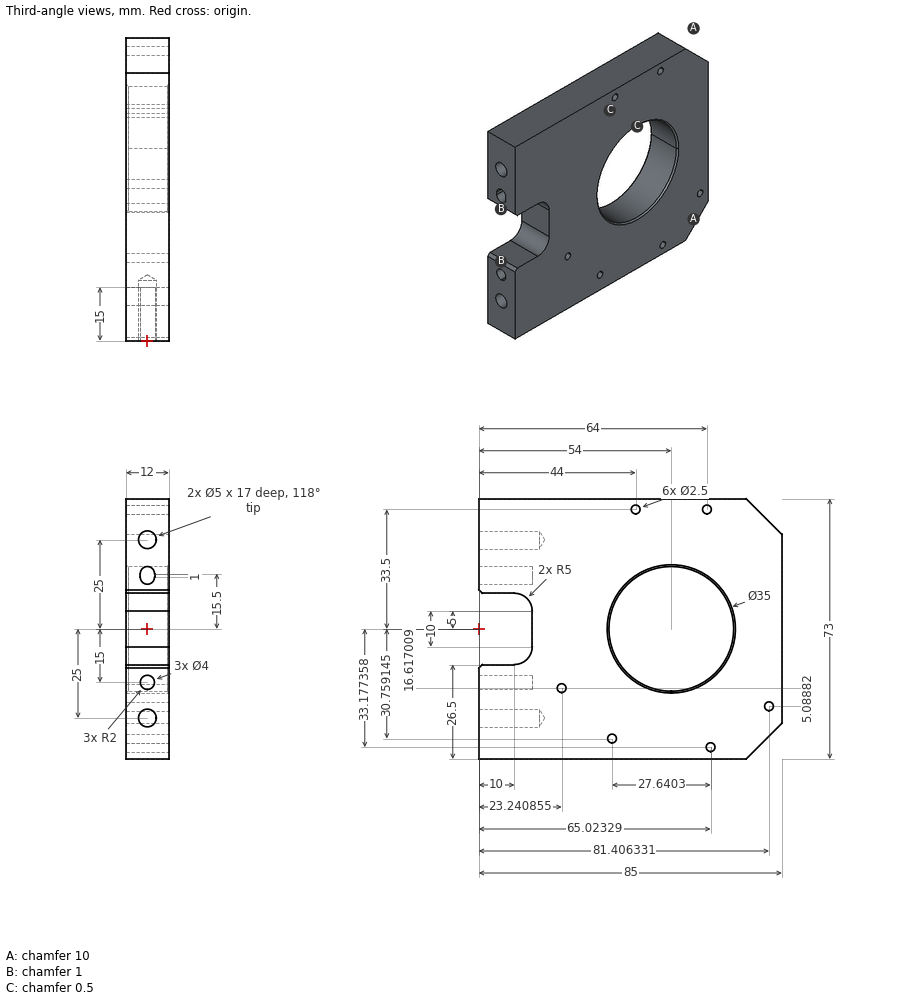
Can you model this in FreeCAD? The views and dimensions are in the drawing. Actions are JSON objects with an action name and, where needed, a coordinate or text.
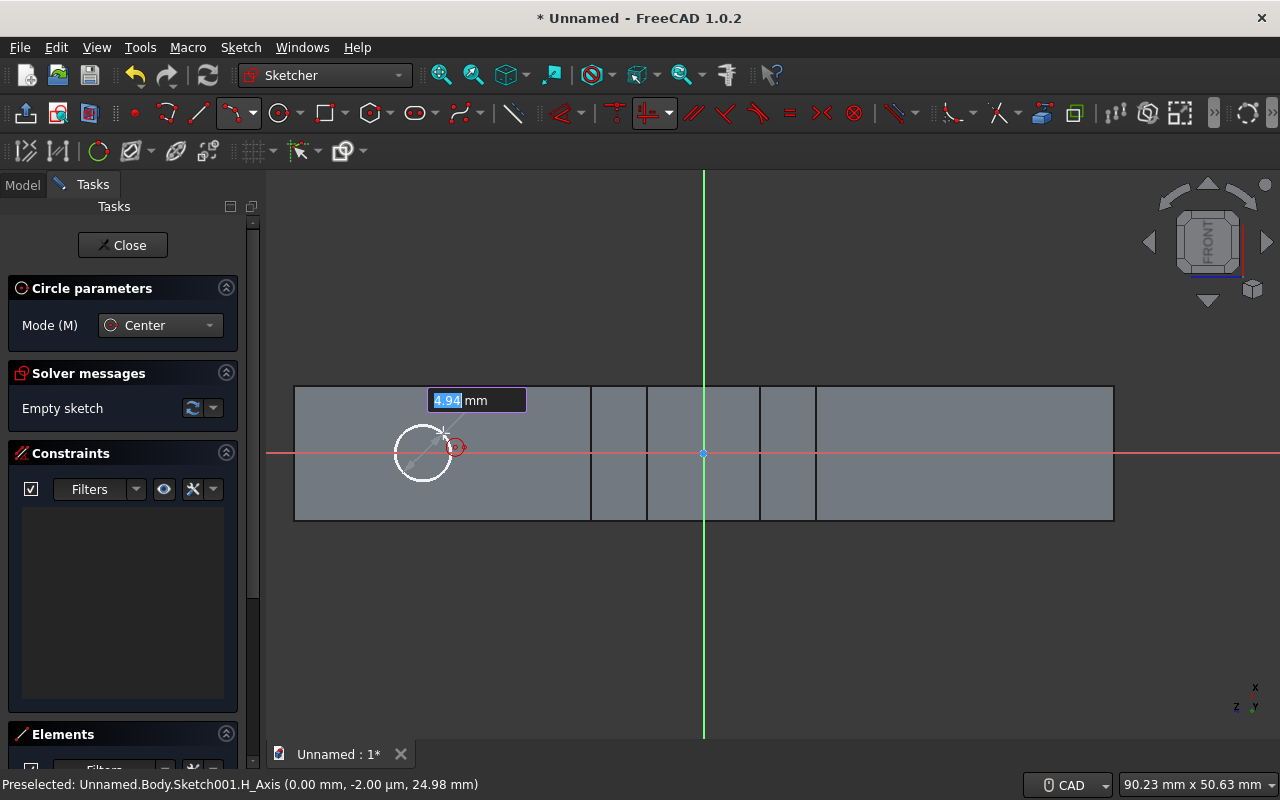
{"action": "type", "text": "5"}
{"action": "key", "text": "Return"}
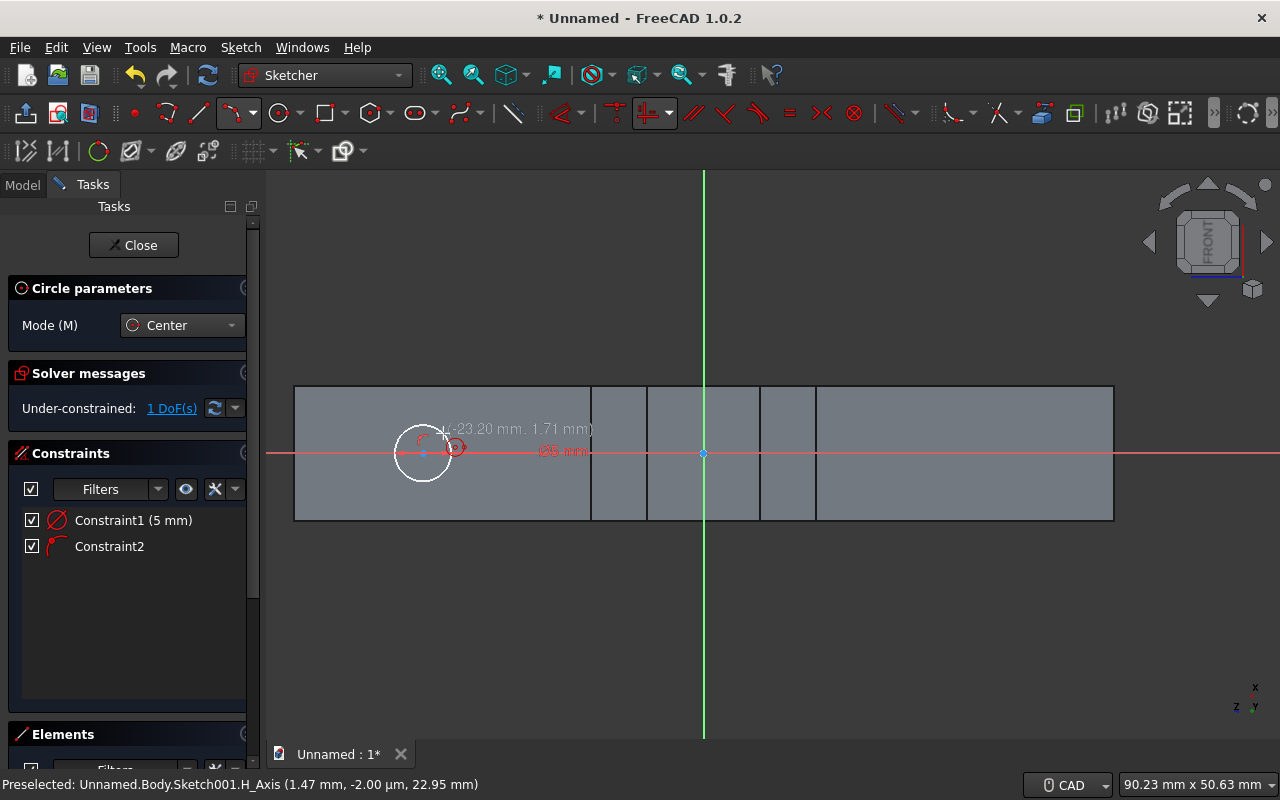
{"action": "left_click", "coordinate": [985, 453]}
{"action": "mouse_move", "coordinate": [1004, 433]}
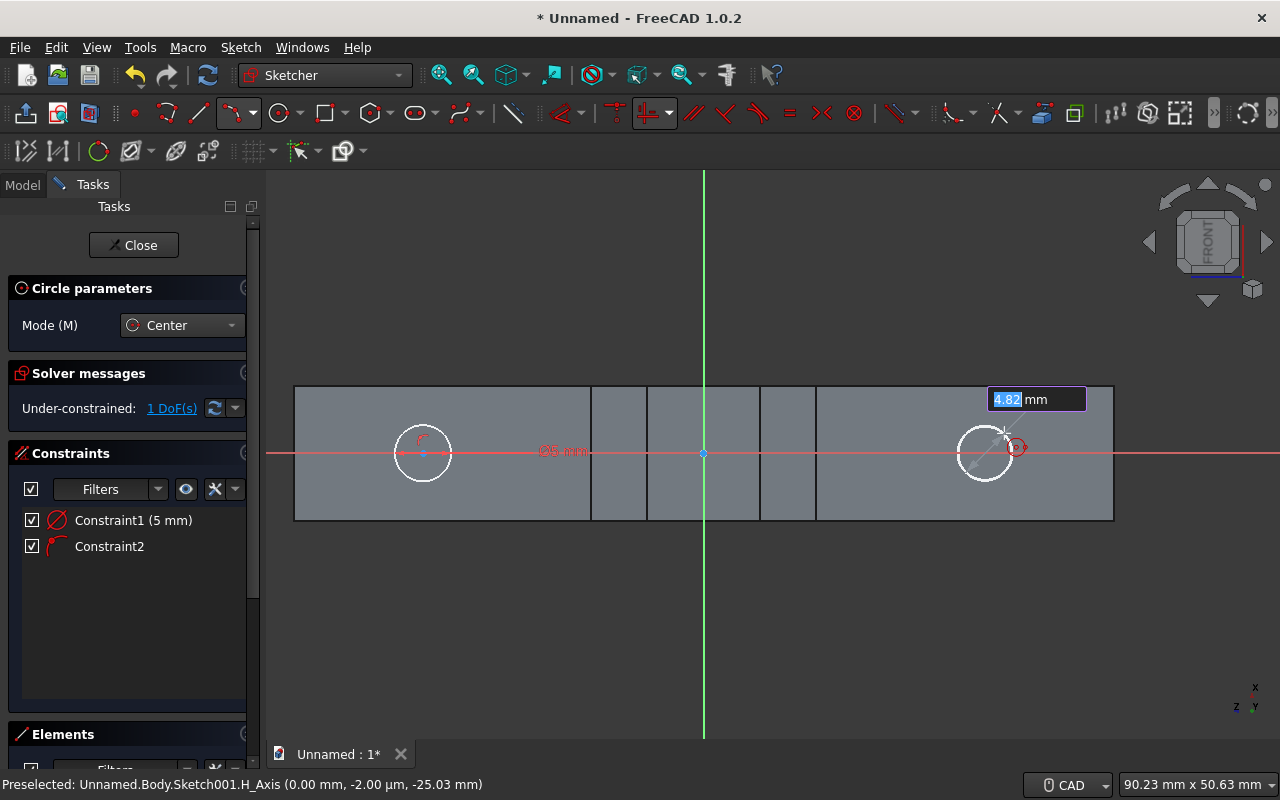
{"action": "type", "text": "5"}
{"action": "key", "text": "Return"}
{"action": "key", "text": "Escape"}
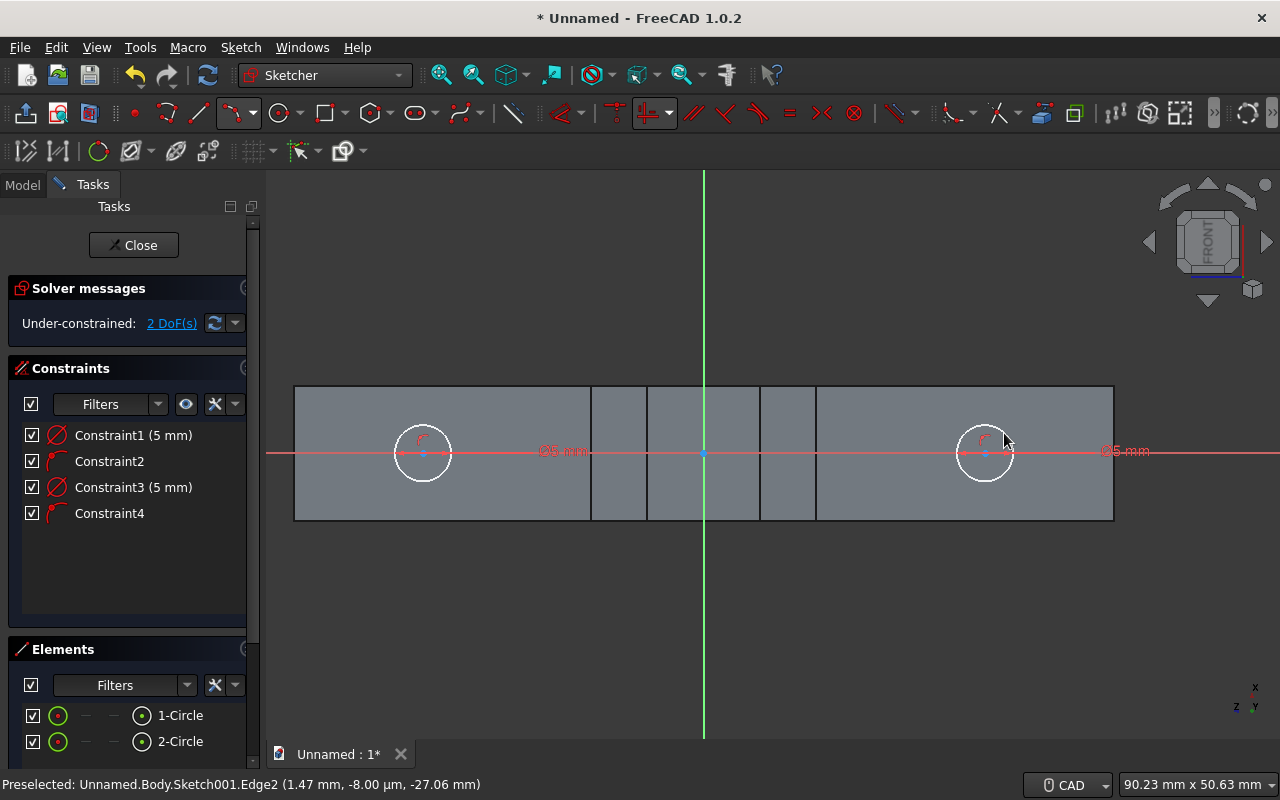
{"action": "left_click", "coordinate": [560, 114]}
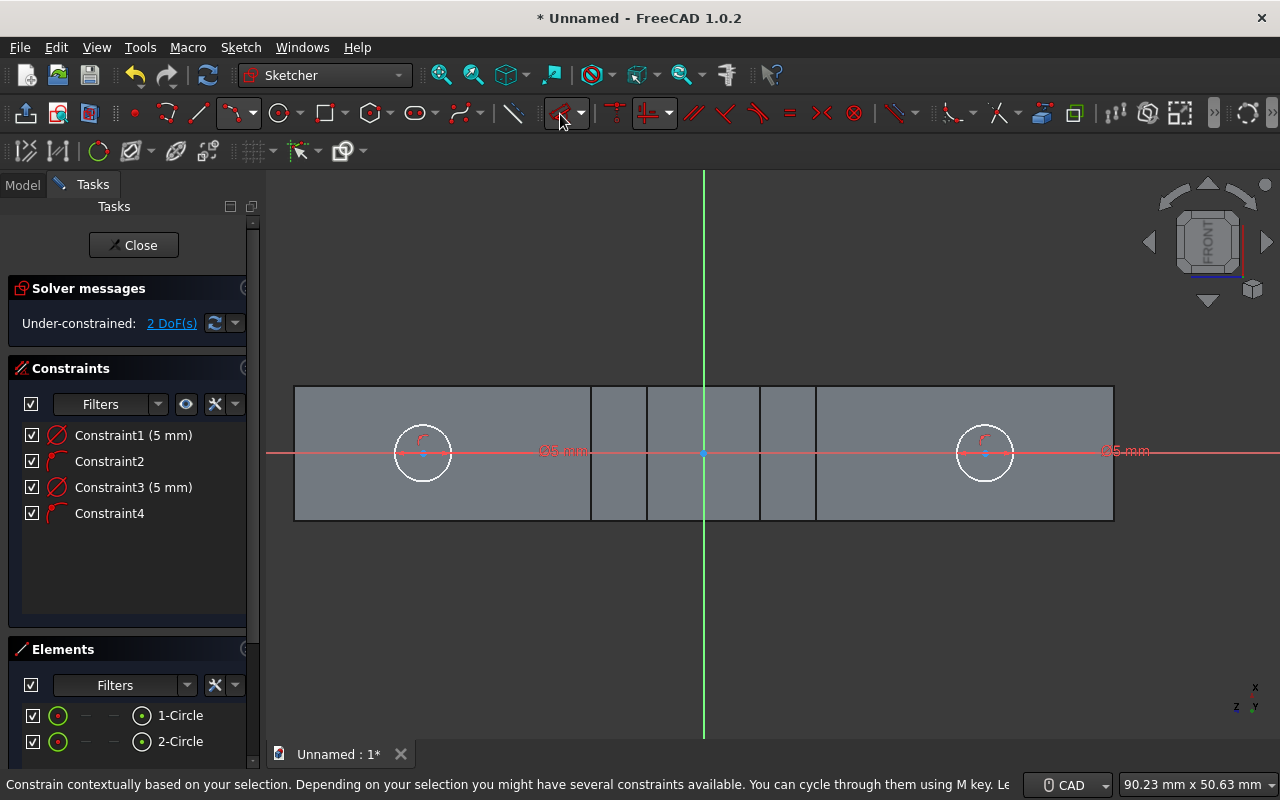
{"action": "left_click", "coordinate": [423, 453]}
{"action": "left_click", "coordinate": [563, 487]}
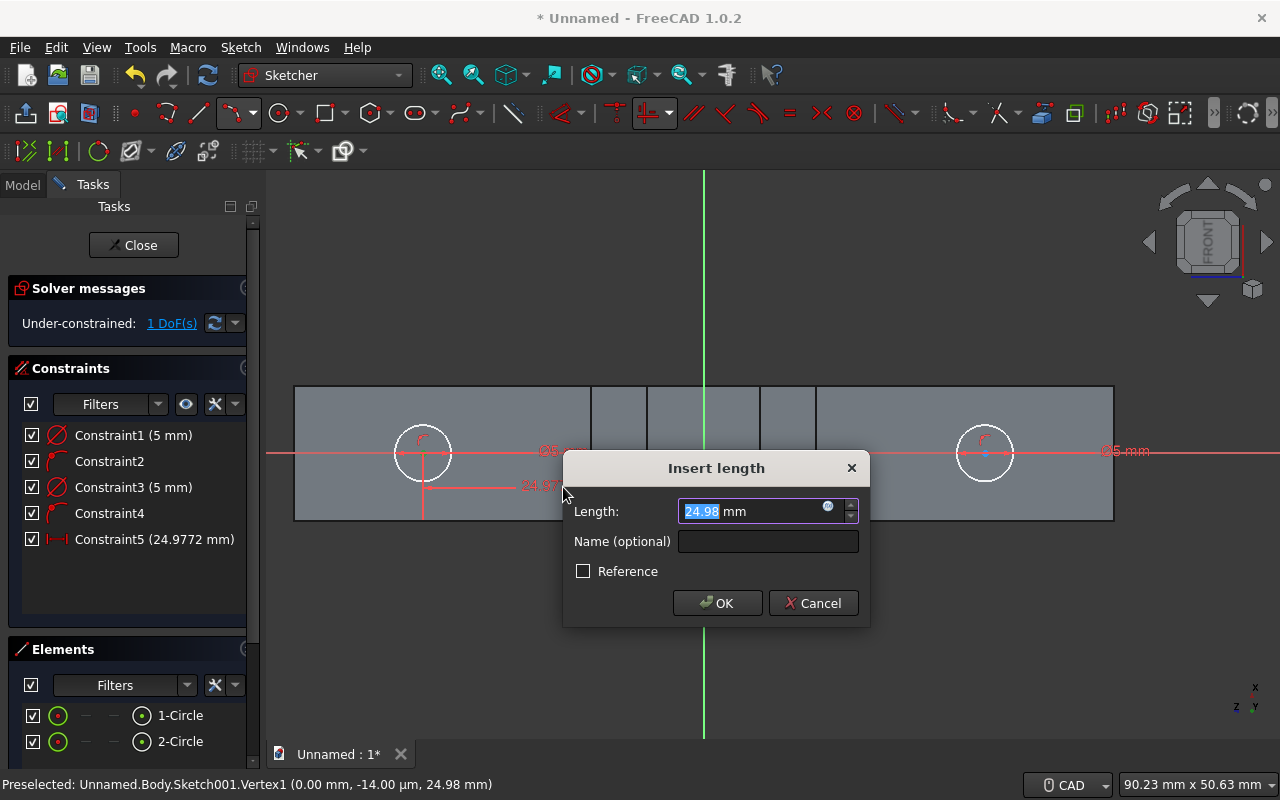
{"action": "type", "text": "25"}
{"action": "key", "text": "Return"}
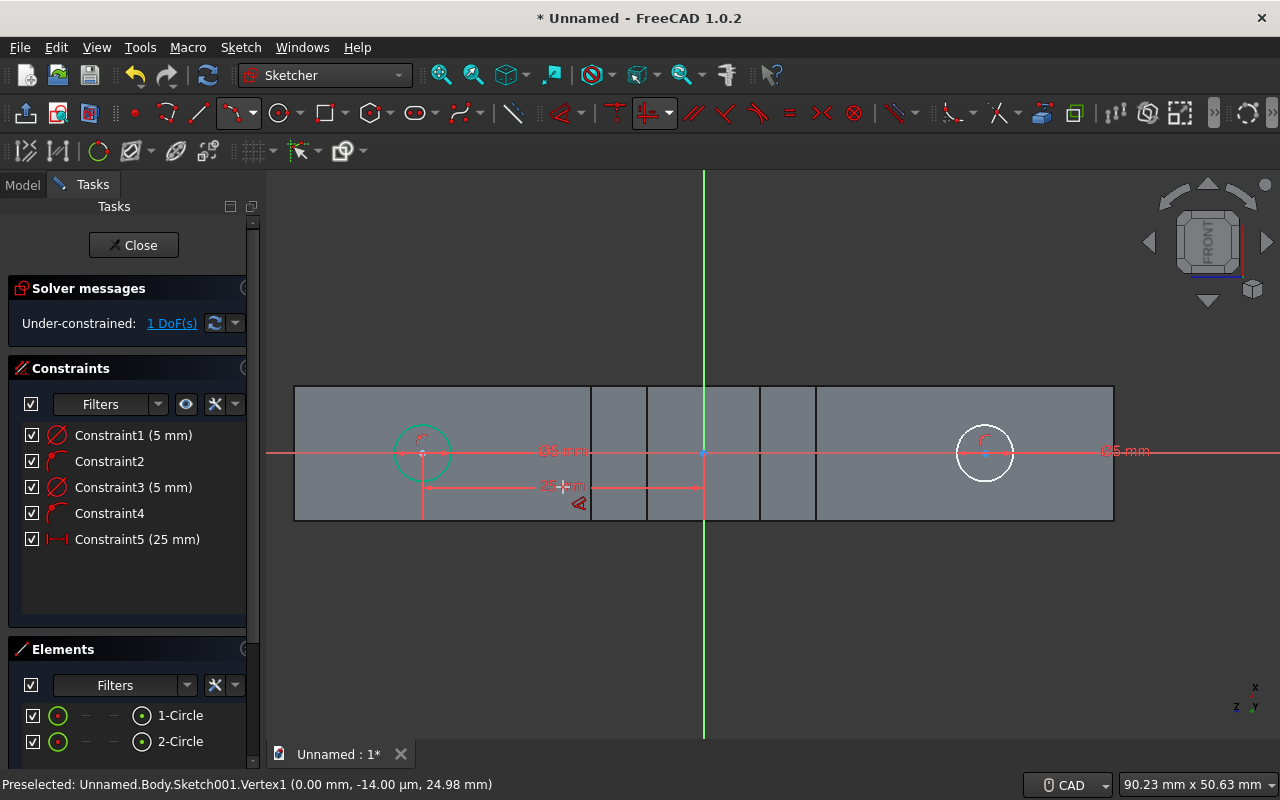
{"action": "left_click", "coordinate": [985, 453]}
{"action": "left_click", "coordinate": [844, 487]}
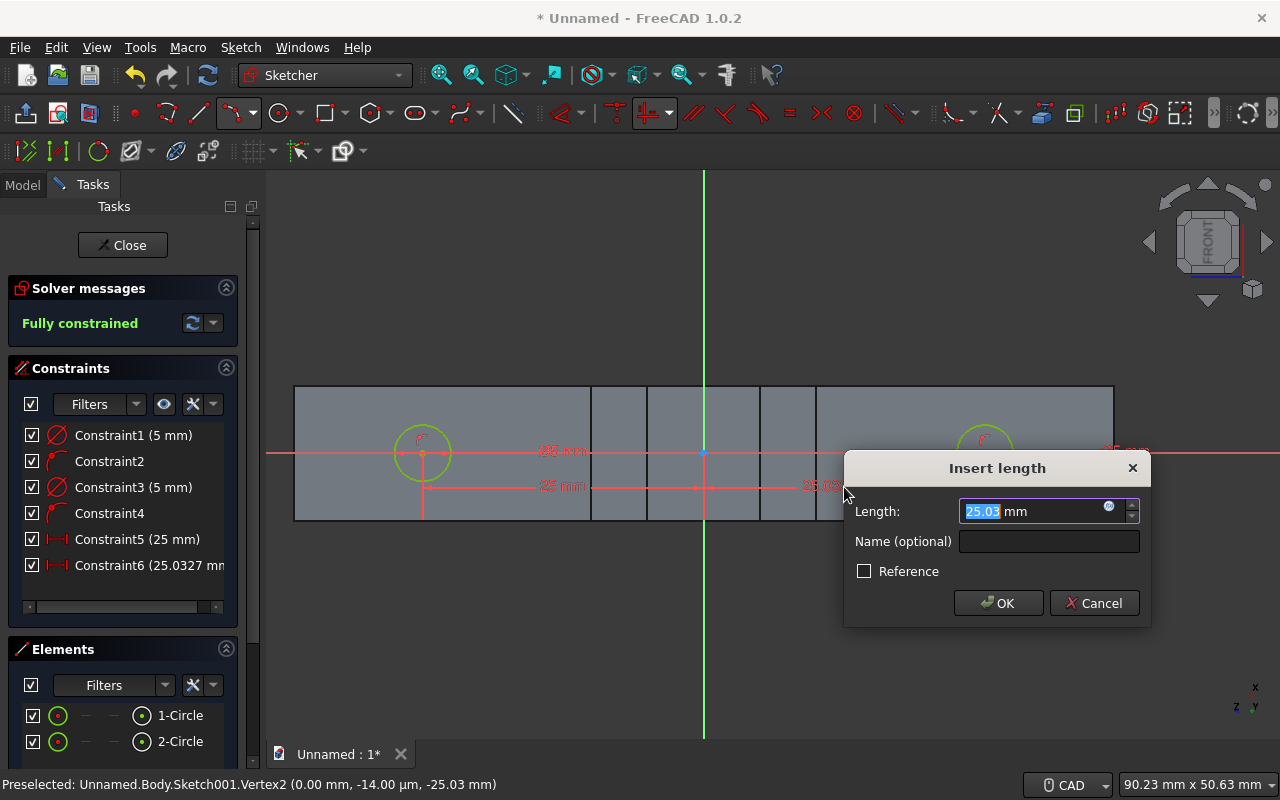
{"action": "type", "text": "25"}
{"action": "key", "text": "Return"}
{"action": "key", "text": "Escape"}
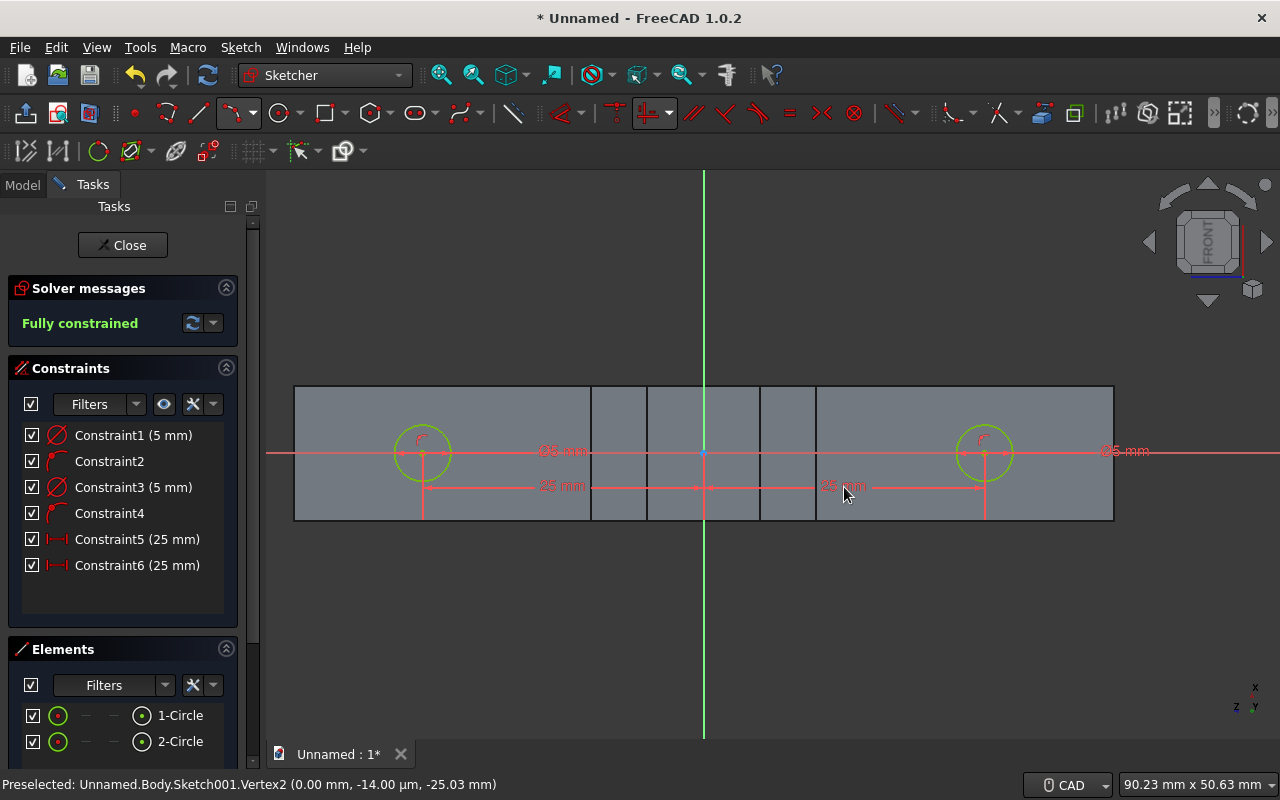
{"action": "left_click", "coordinate": [123, 245]}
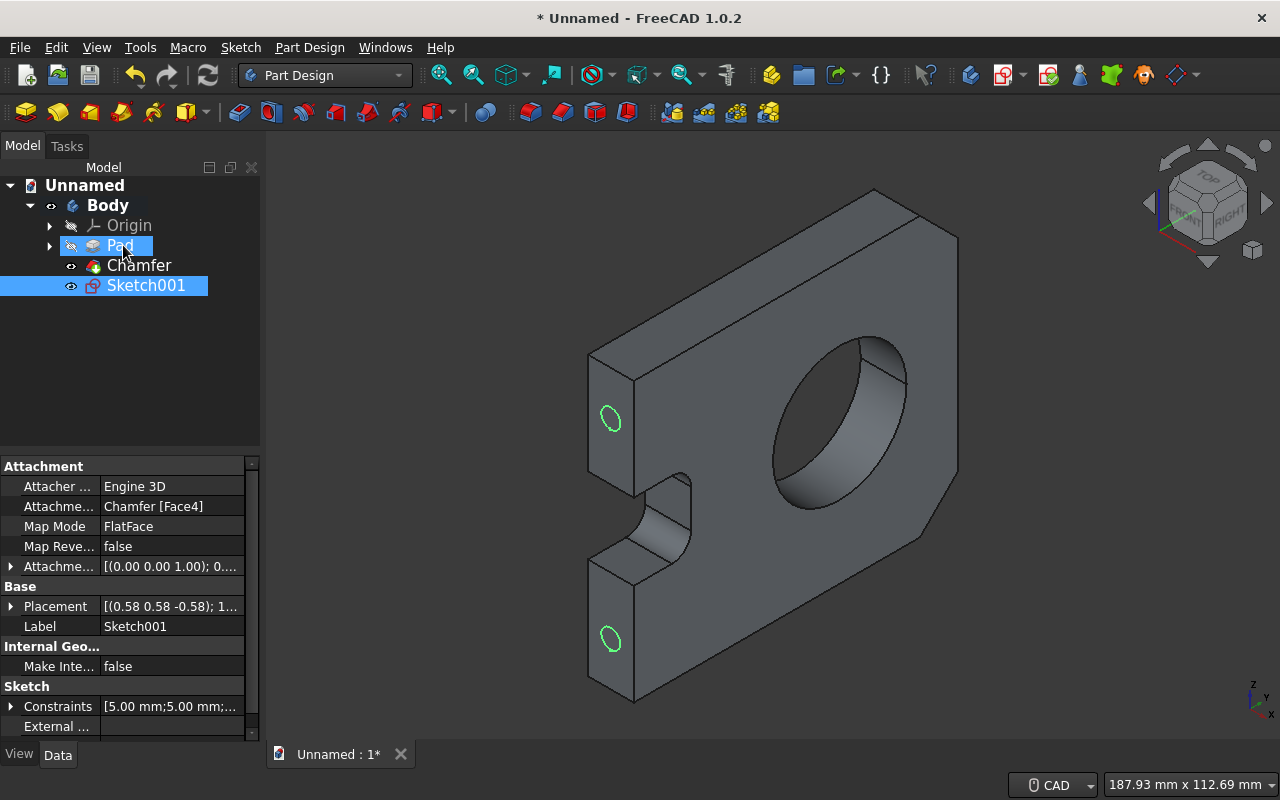
{"action": "left_click", "coordinate": [272, 112]}